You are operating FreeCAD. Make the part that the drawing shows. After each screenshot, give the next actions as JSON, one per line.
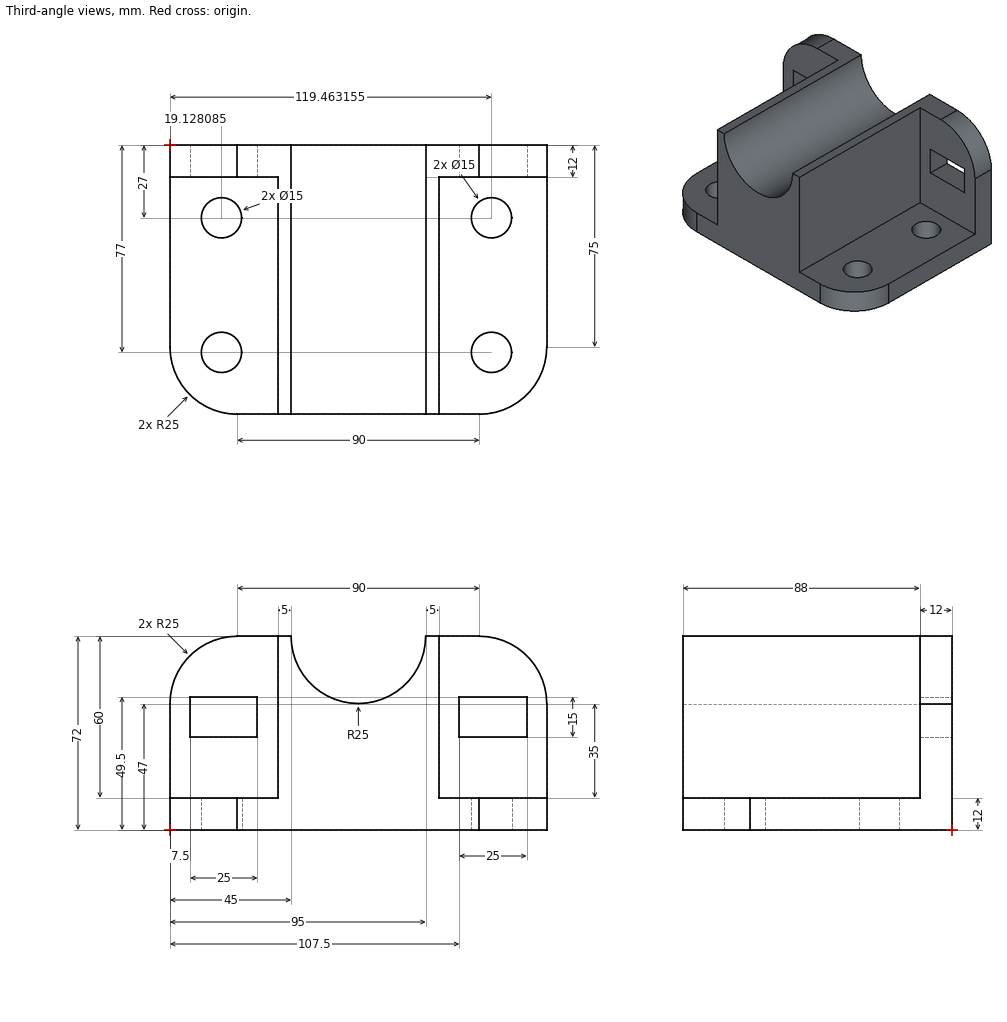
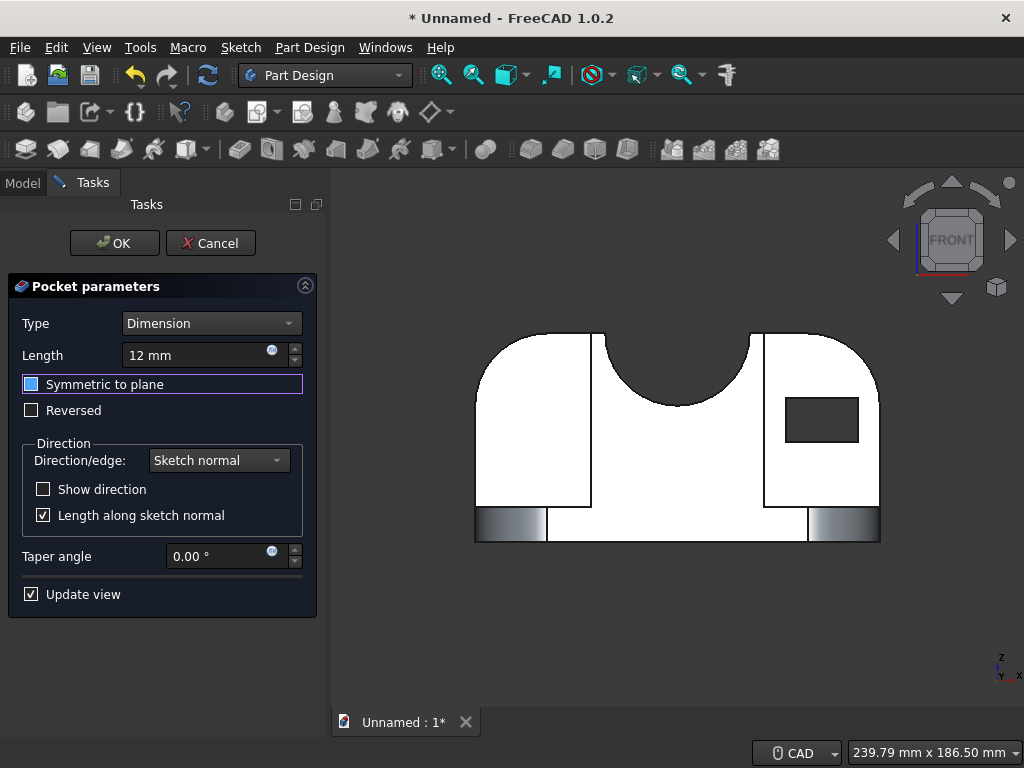
{"action": "left_click", "coordinate": [115, 243]}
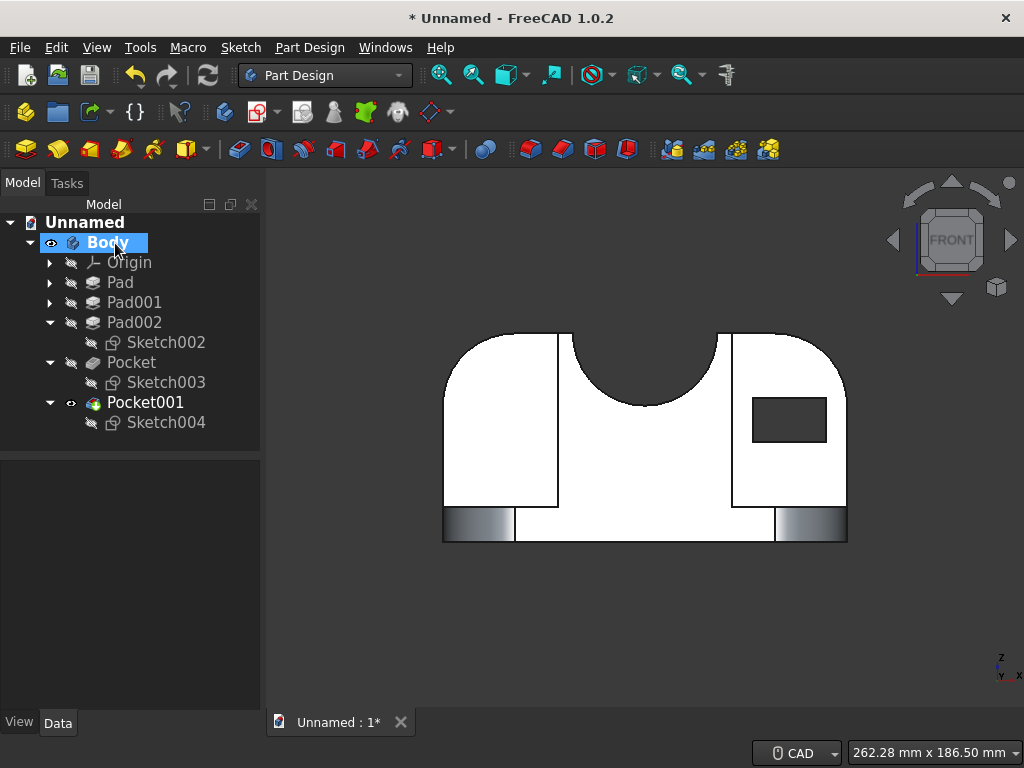
{"action": "left_click", "coordinate": [500, 419]}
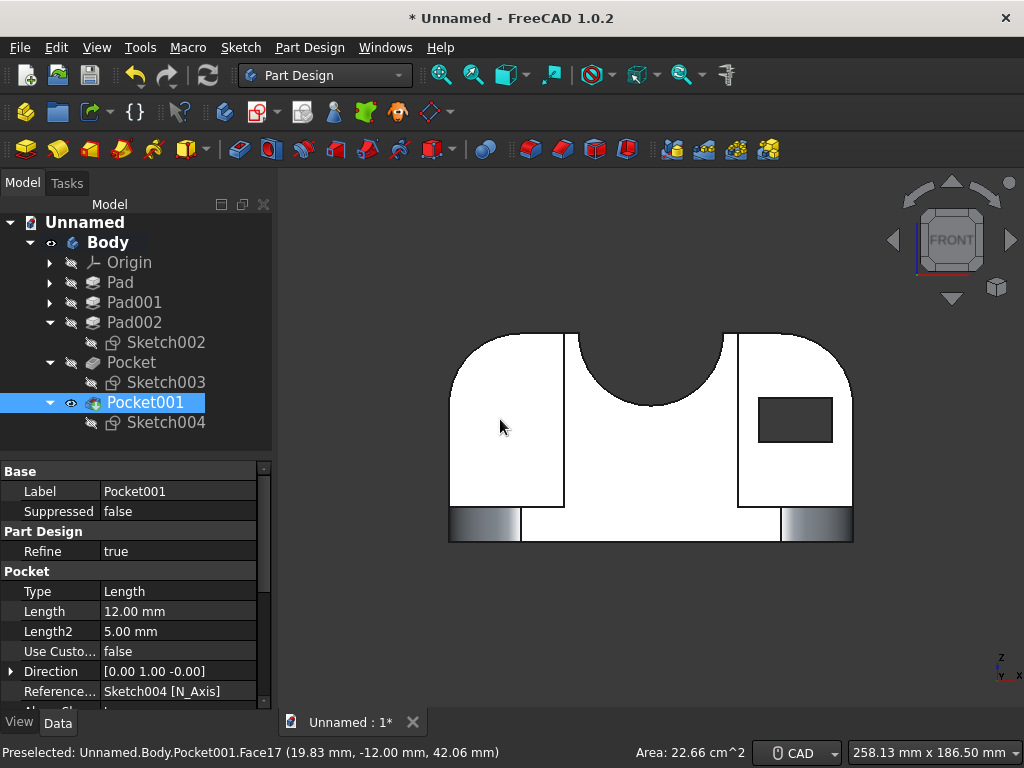
{"action": "left_click", "coordinate": [258, 112]}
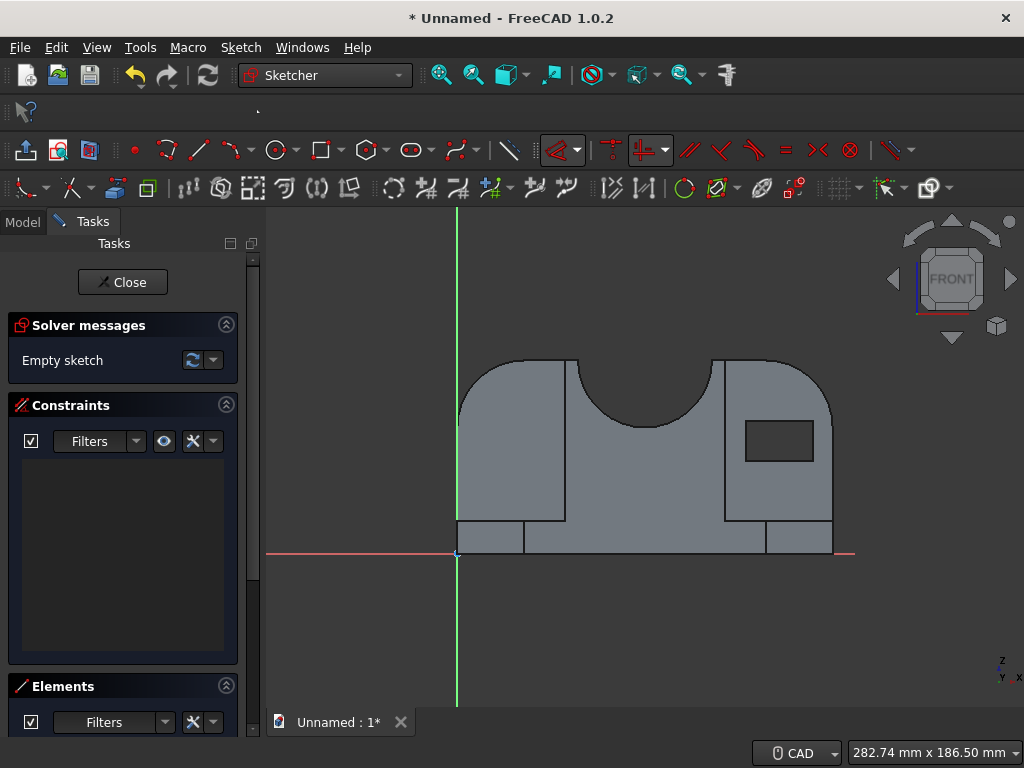
{"action": "key", "text": "q s"}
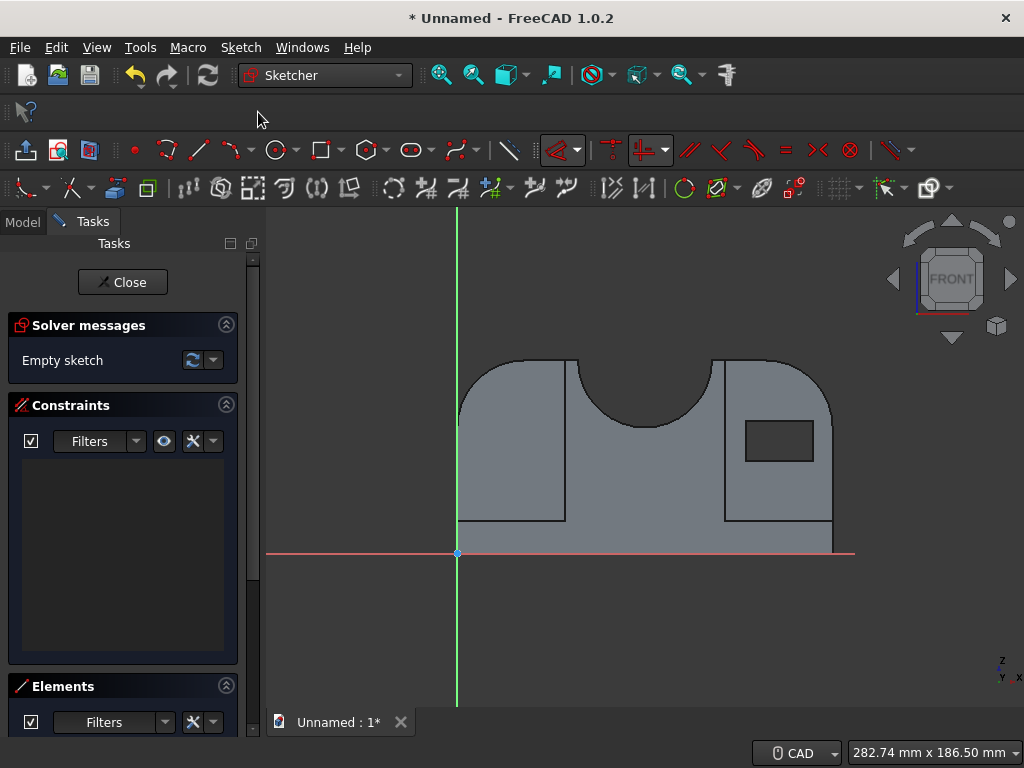
{"action": "scroll", "coordinate": [439, 512], "scroll_direction": "up", "scroll_amount": 4}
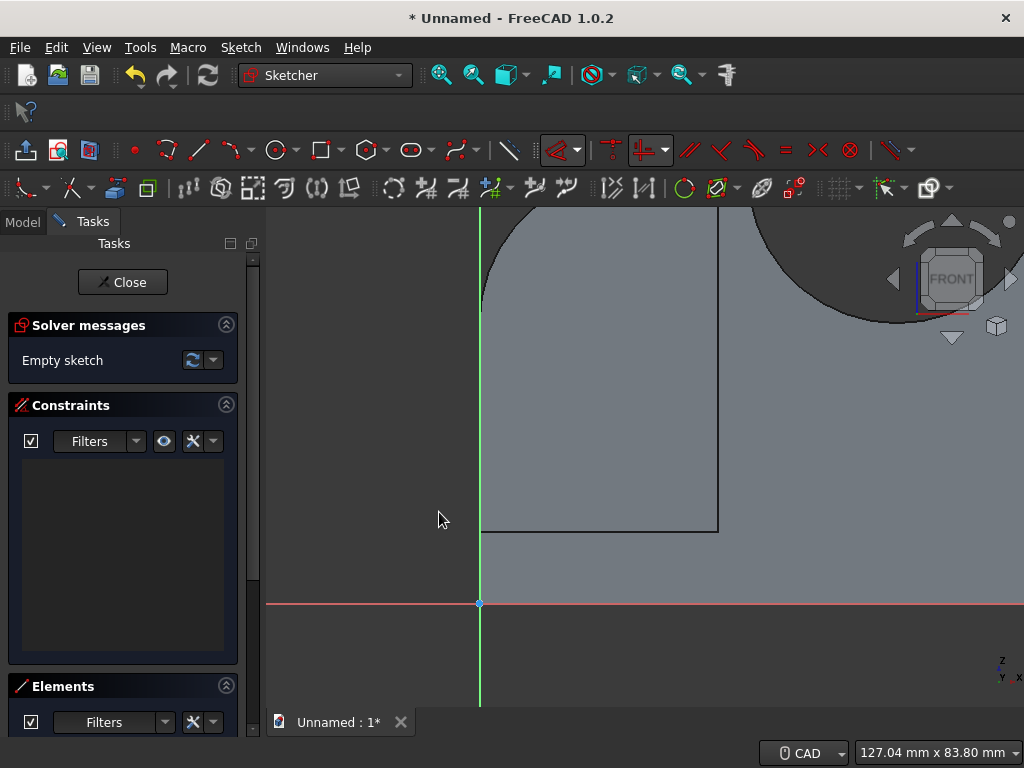
{"action": "key", "text": "g r"}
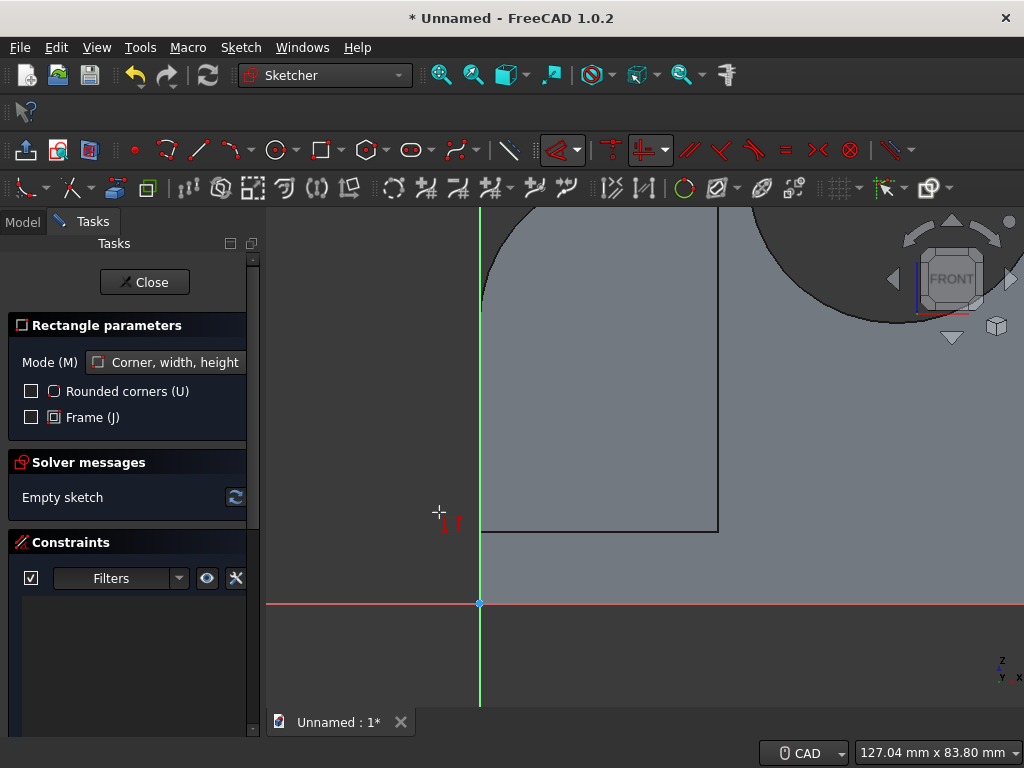
{"action": "left_click", "coordinate": [524, 308]}
{"action": "left_click", "coordinate": [673, 398]}
{"action": "key", "text": "Escape"}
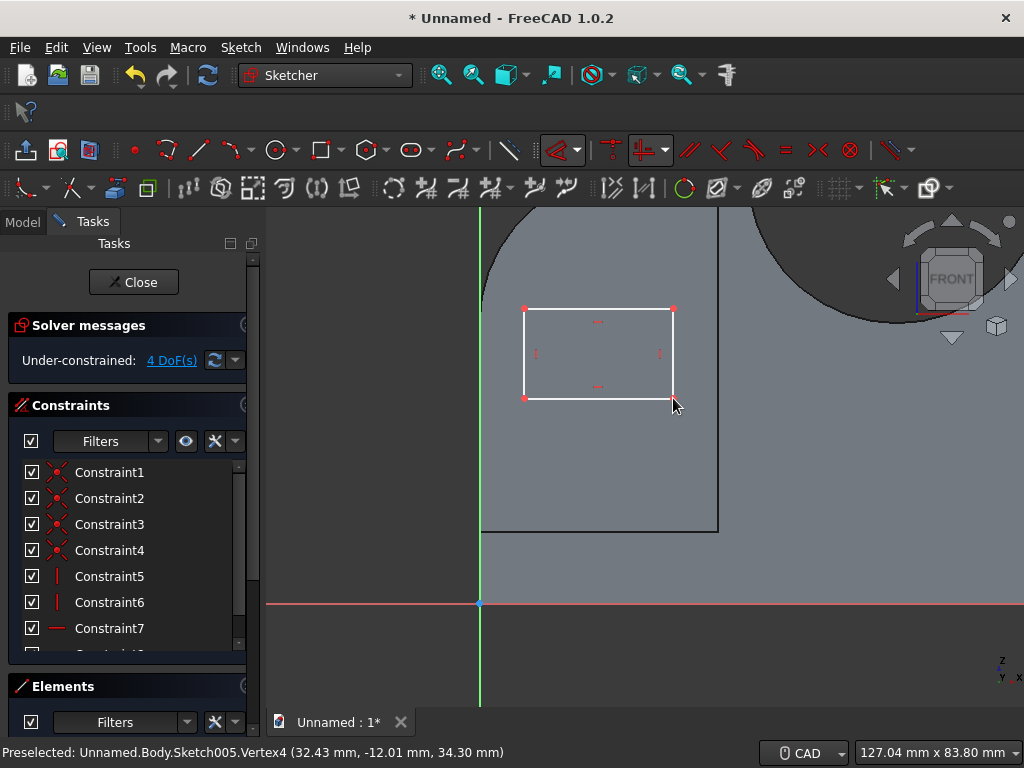
{"action": "left_click", "coordinate": [524, 336]}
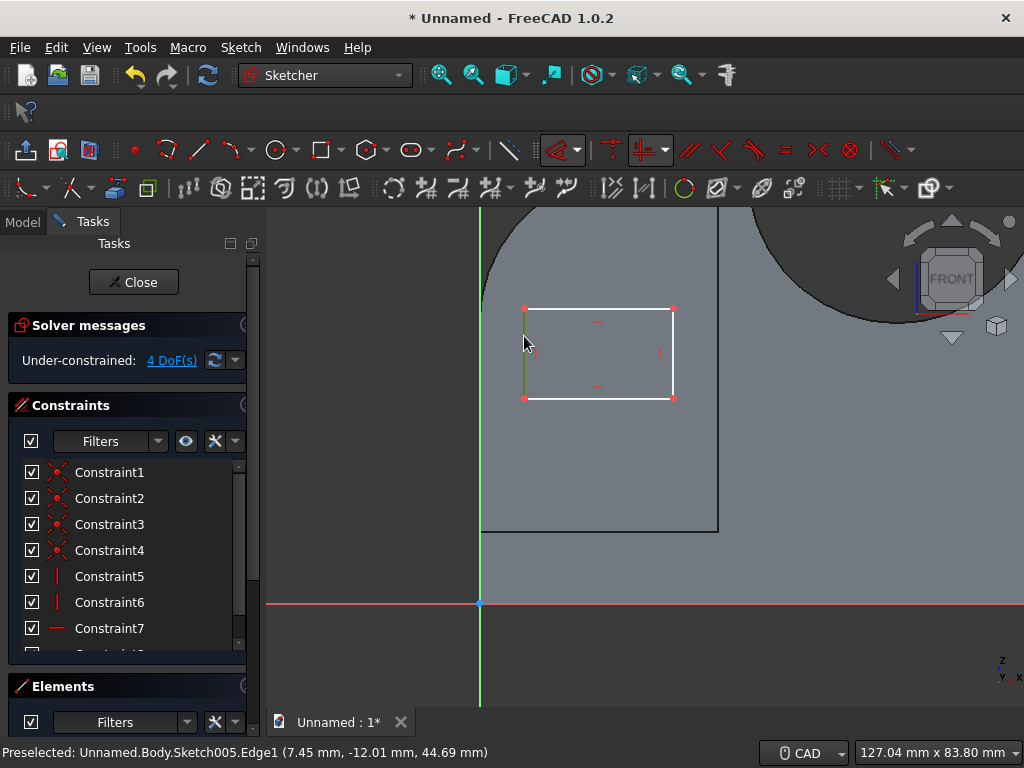
{"action": "key", "text": "i"}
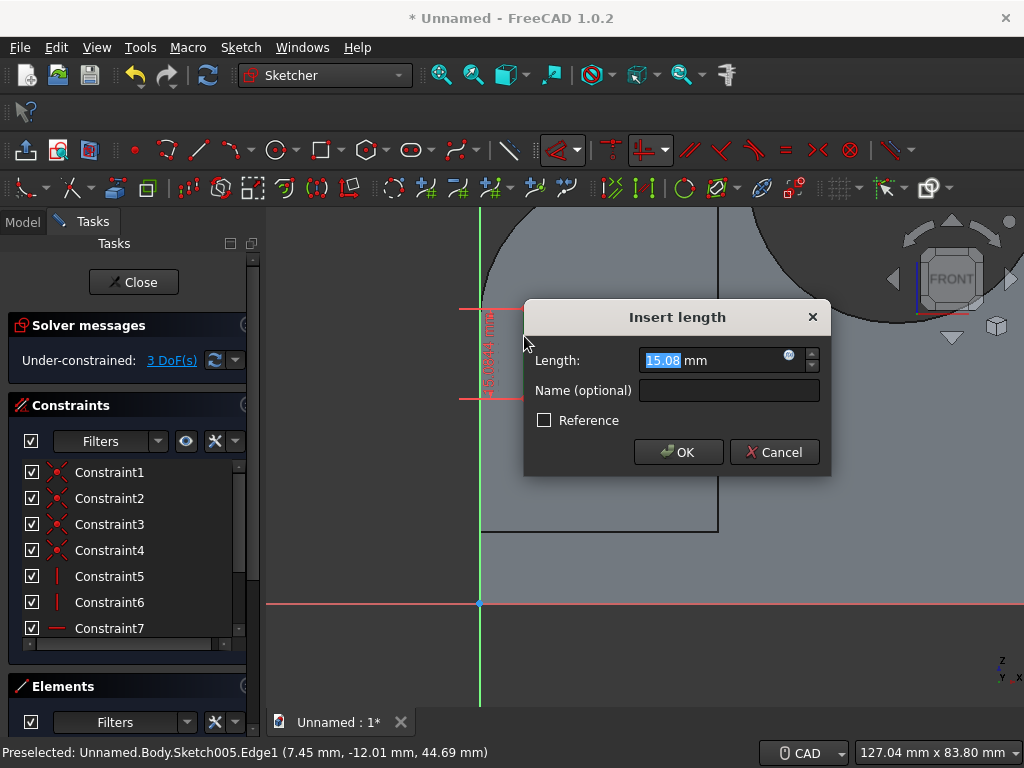
{"action": "type", "text": "15"}
{"action": "key", "text": "Return"}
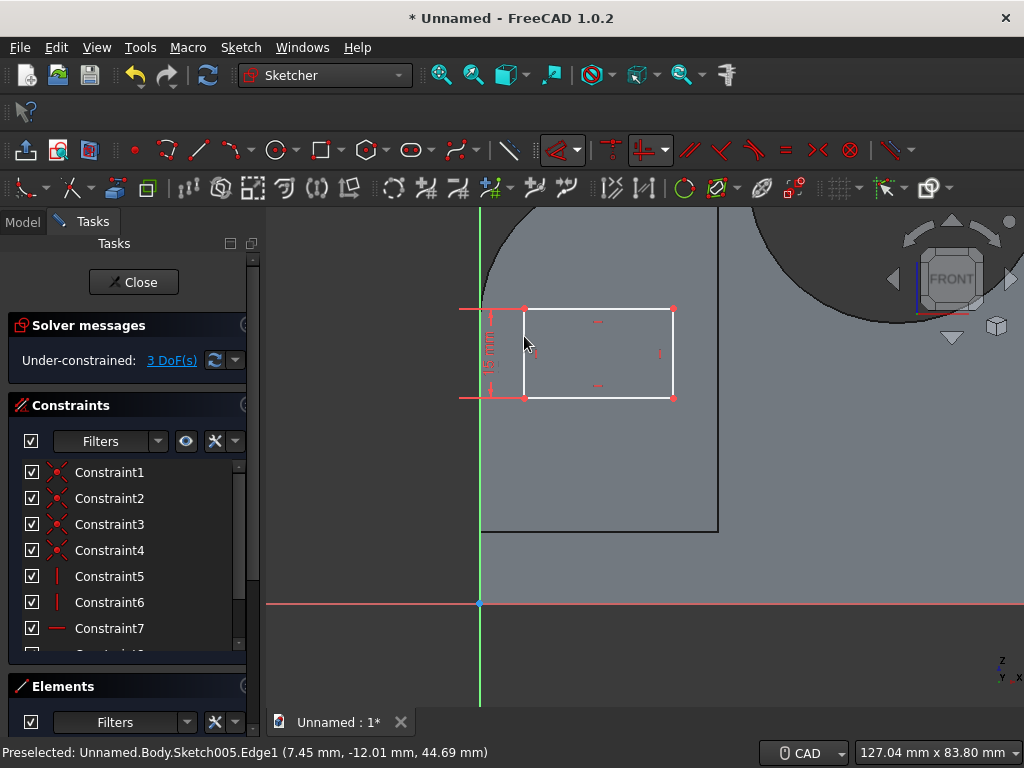
{"action": "left_click", "coordinate": [569, 398]}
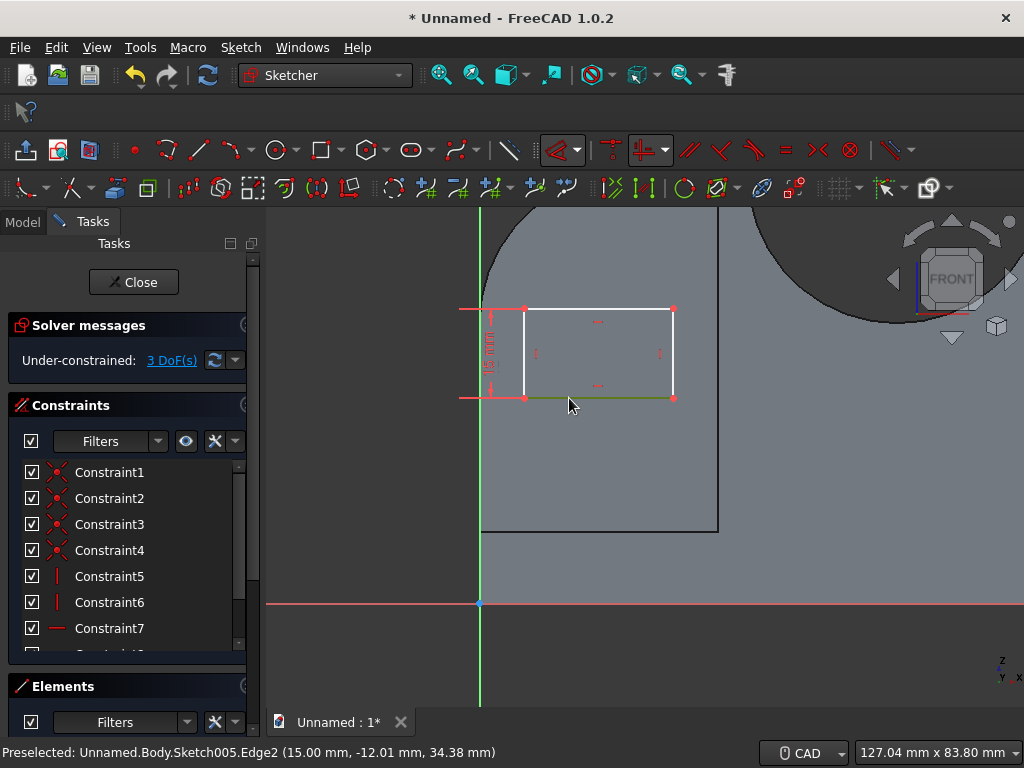
{"action": "key", "text": "l"}